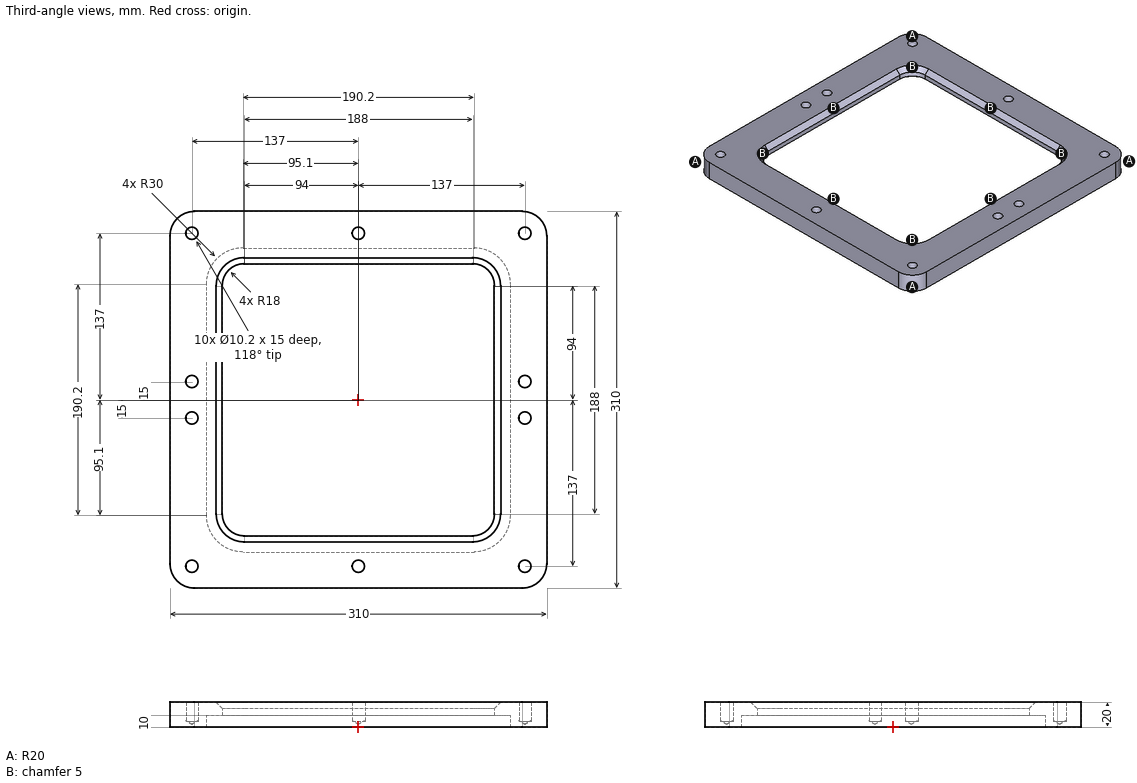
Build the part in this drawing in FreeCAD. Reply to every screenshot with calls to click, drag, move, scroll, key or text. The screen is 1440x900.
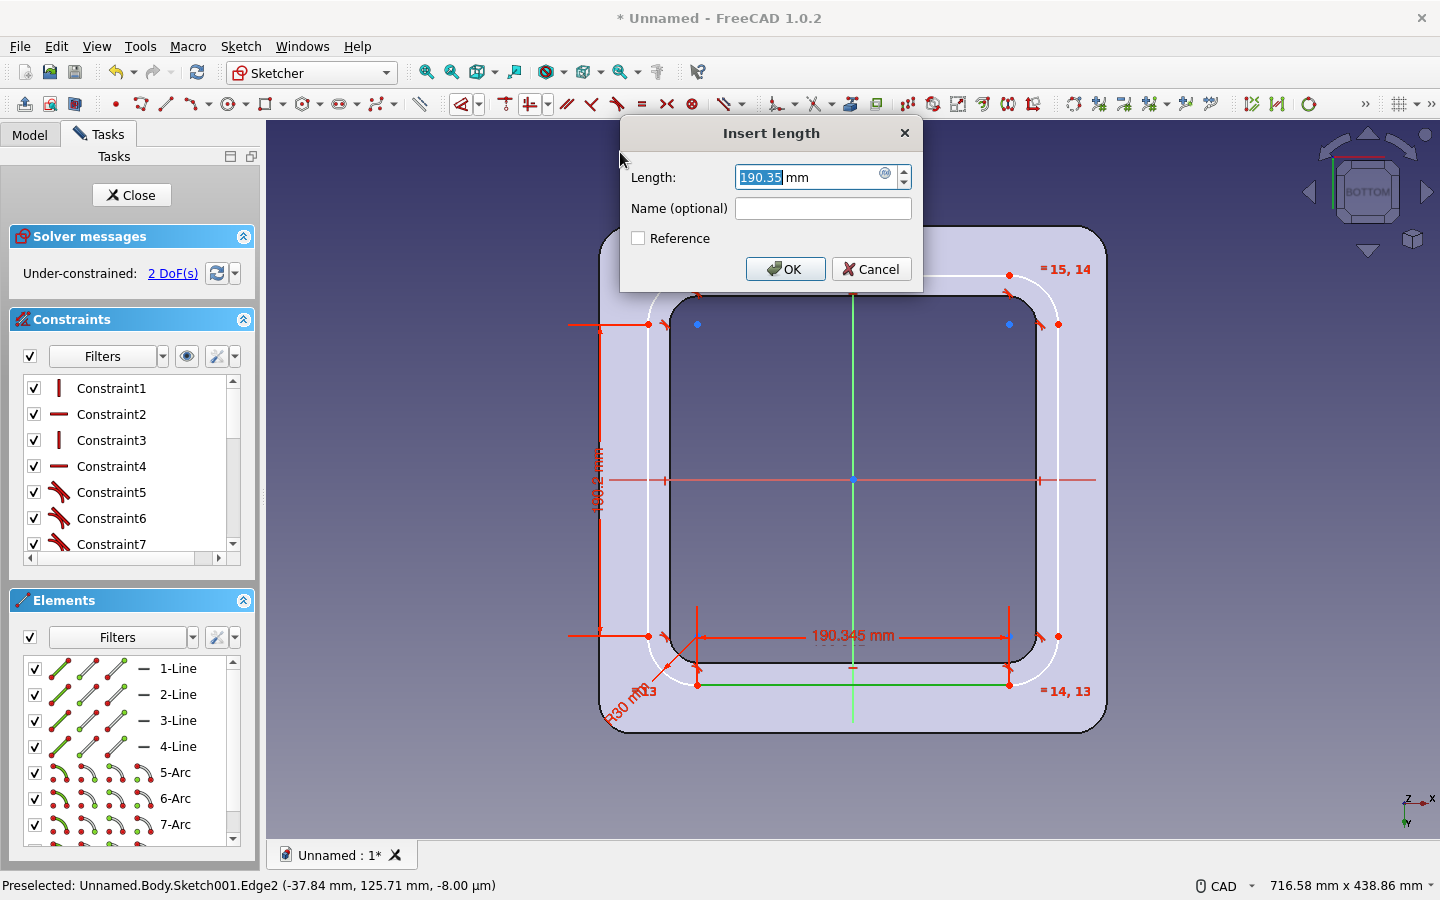
text(190.2)
key(Return)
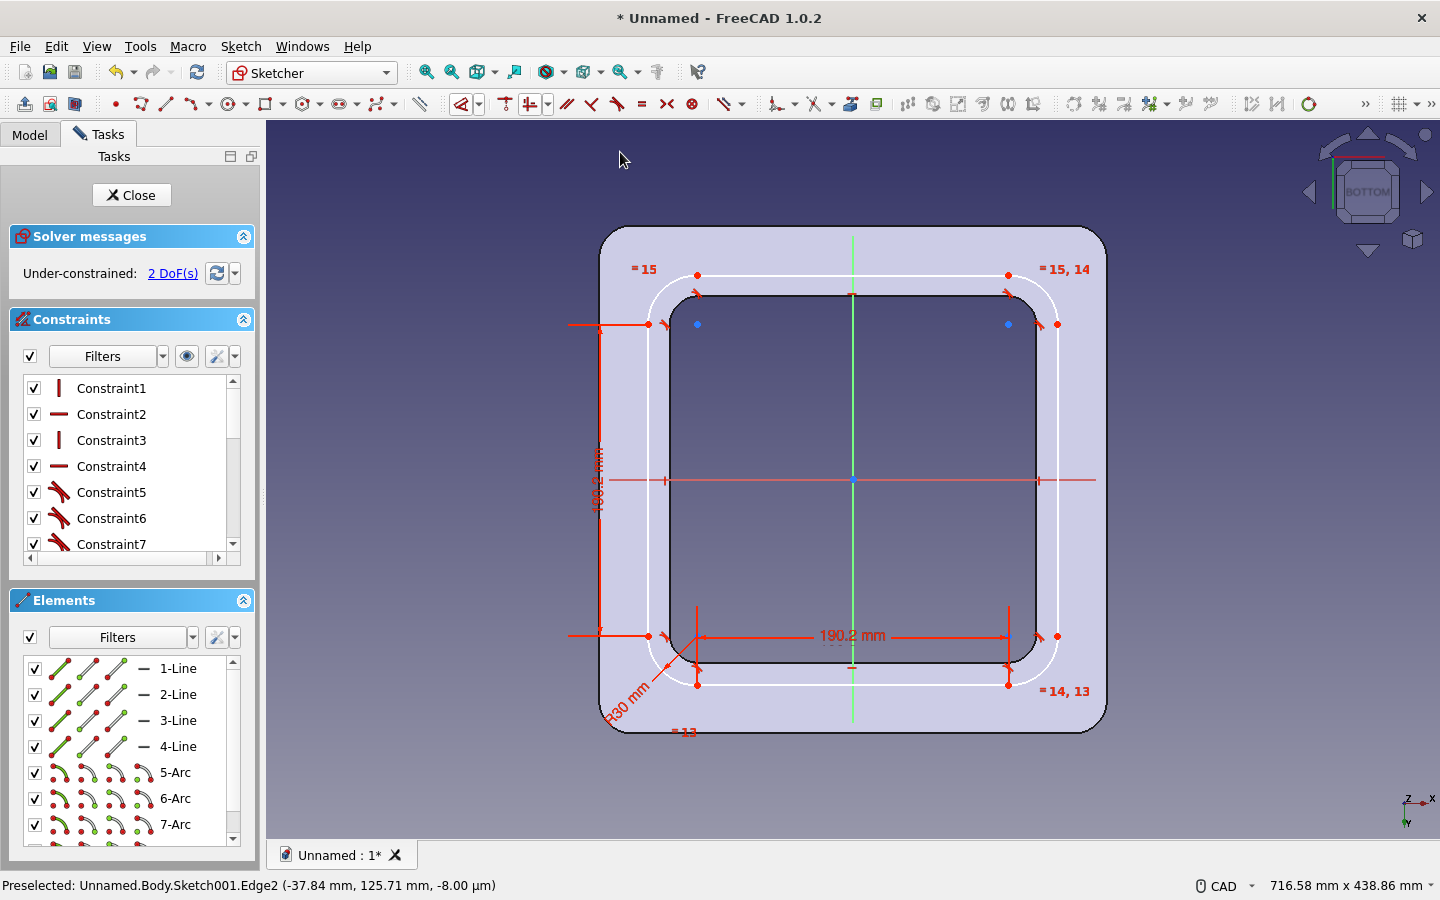
click(648, 325)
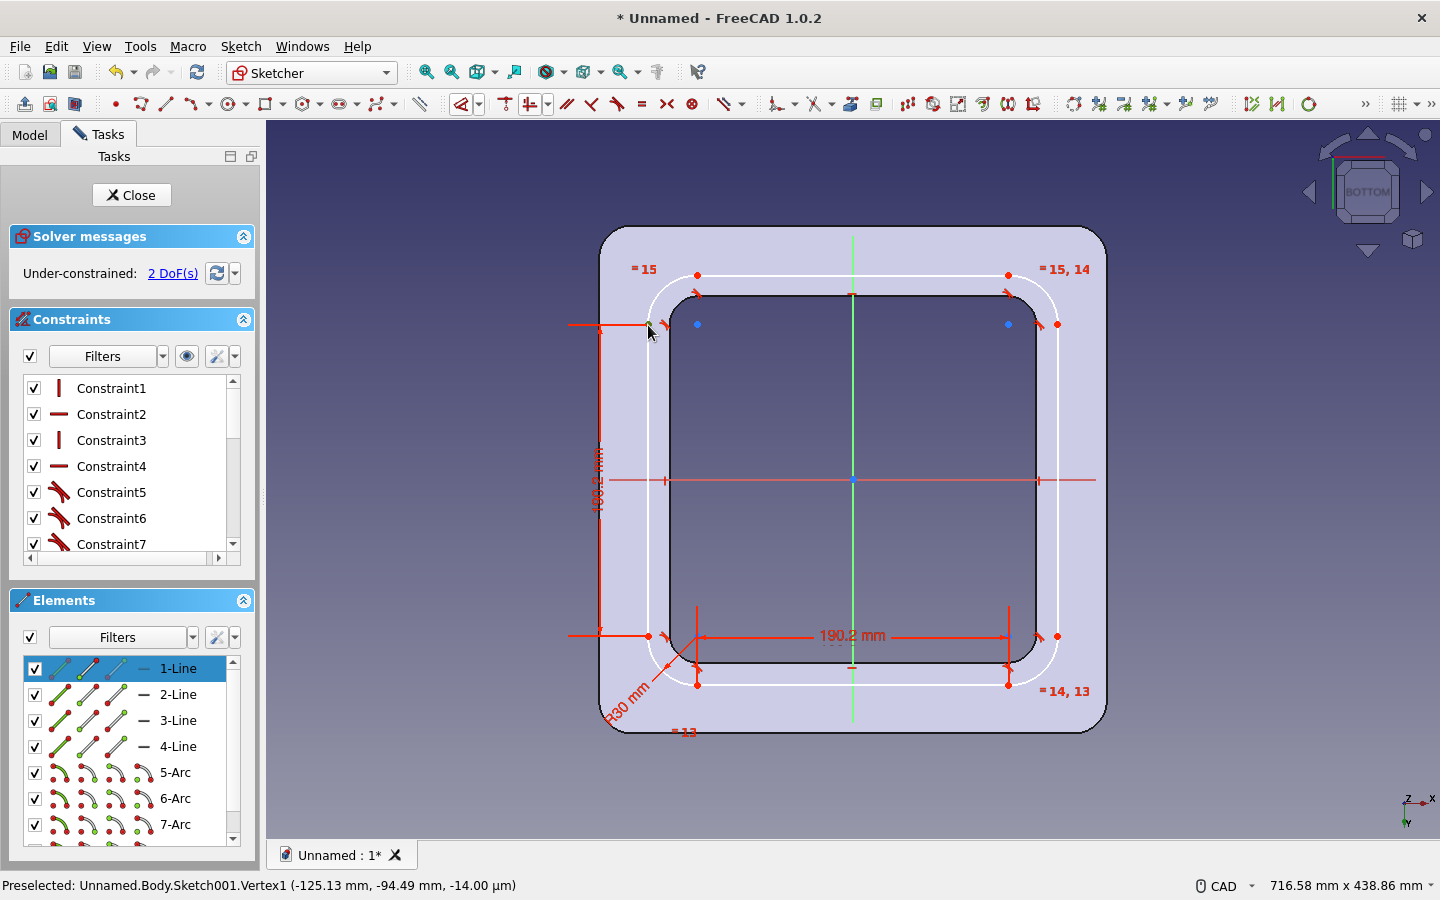
click(478, 104)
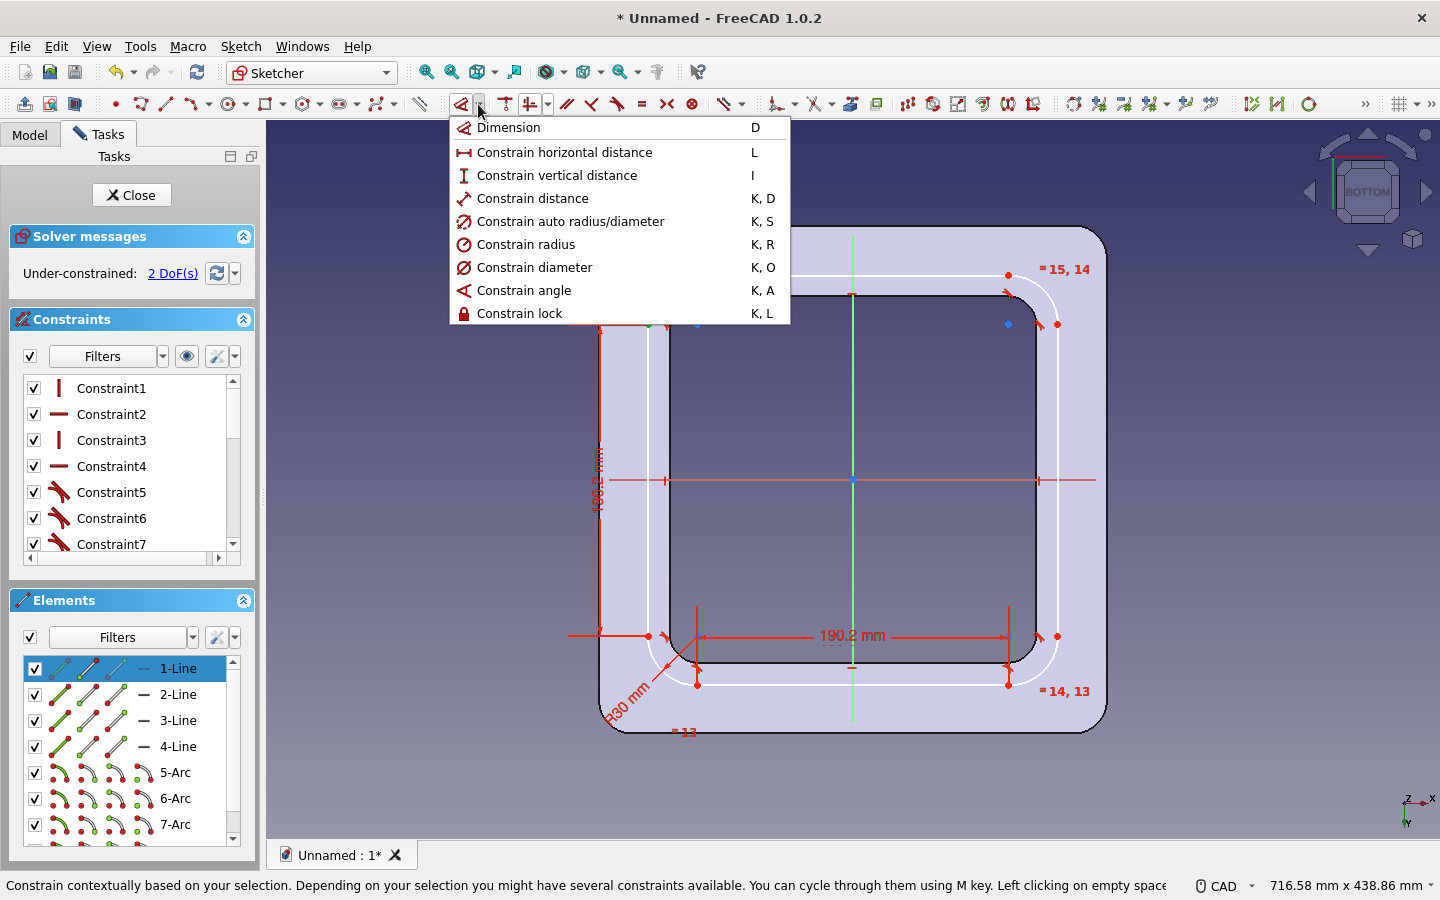
click(620, 176)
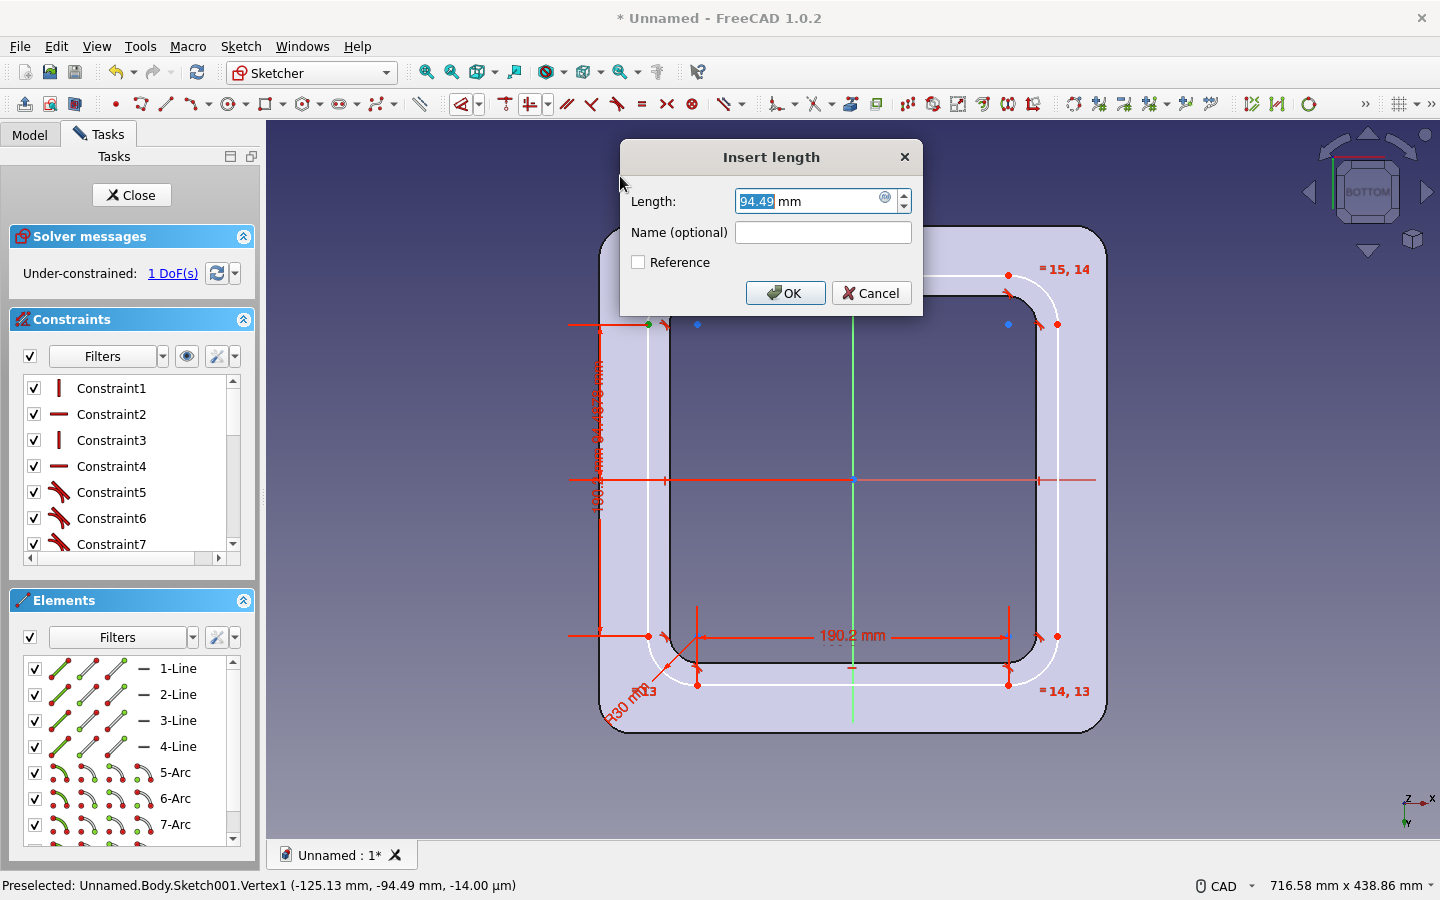
text(95.1)
key(Return)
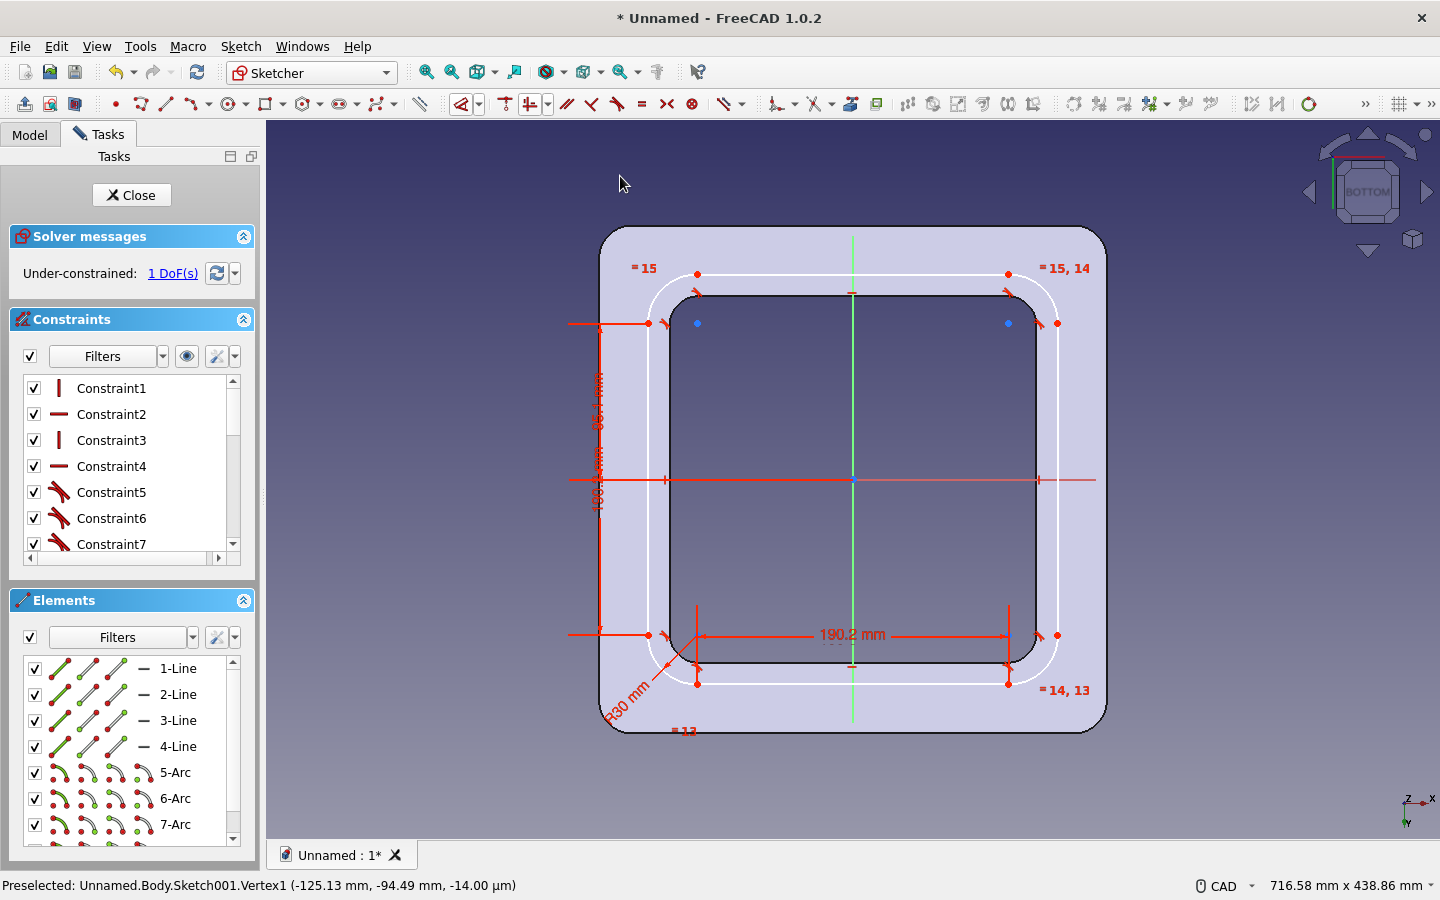
click(697, 684)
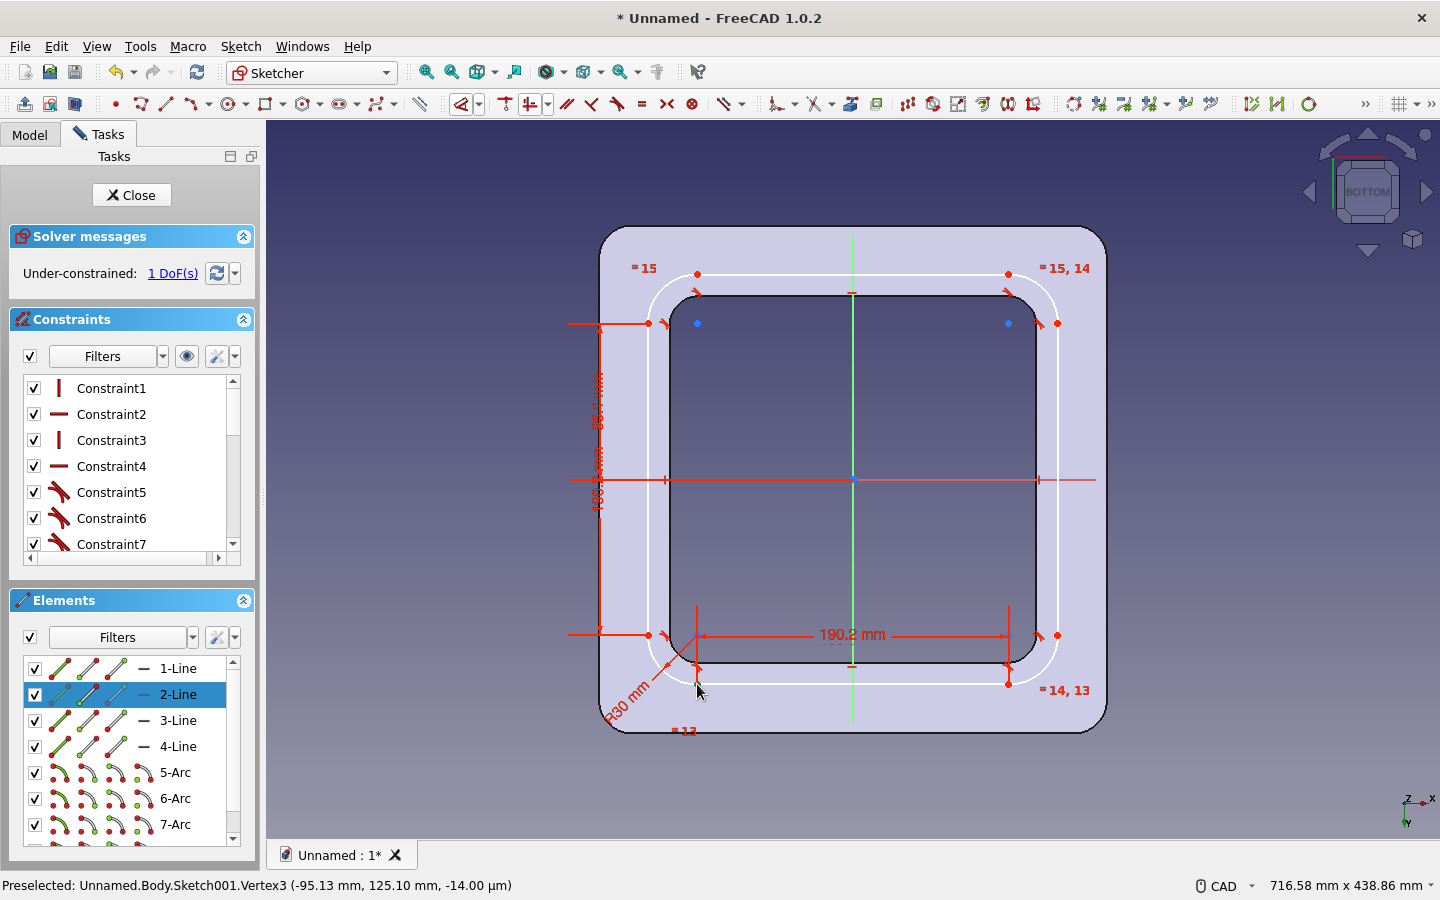
click(478, 104)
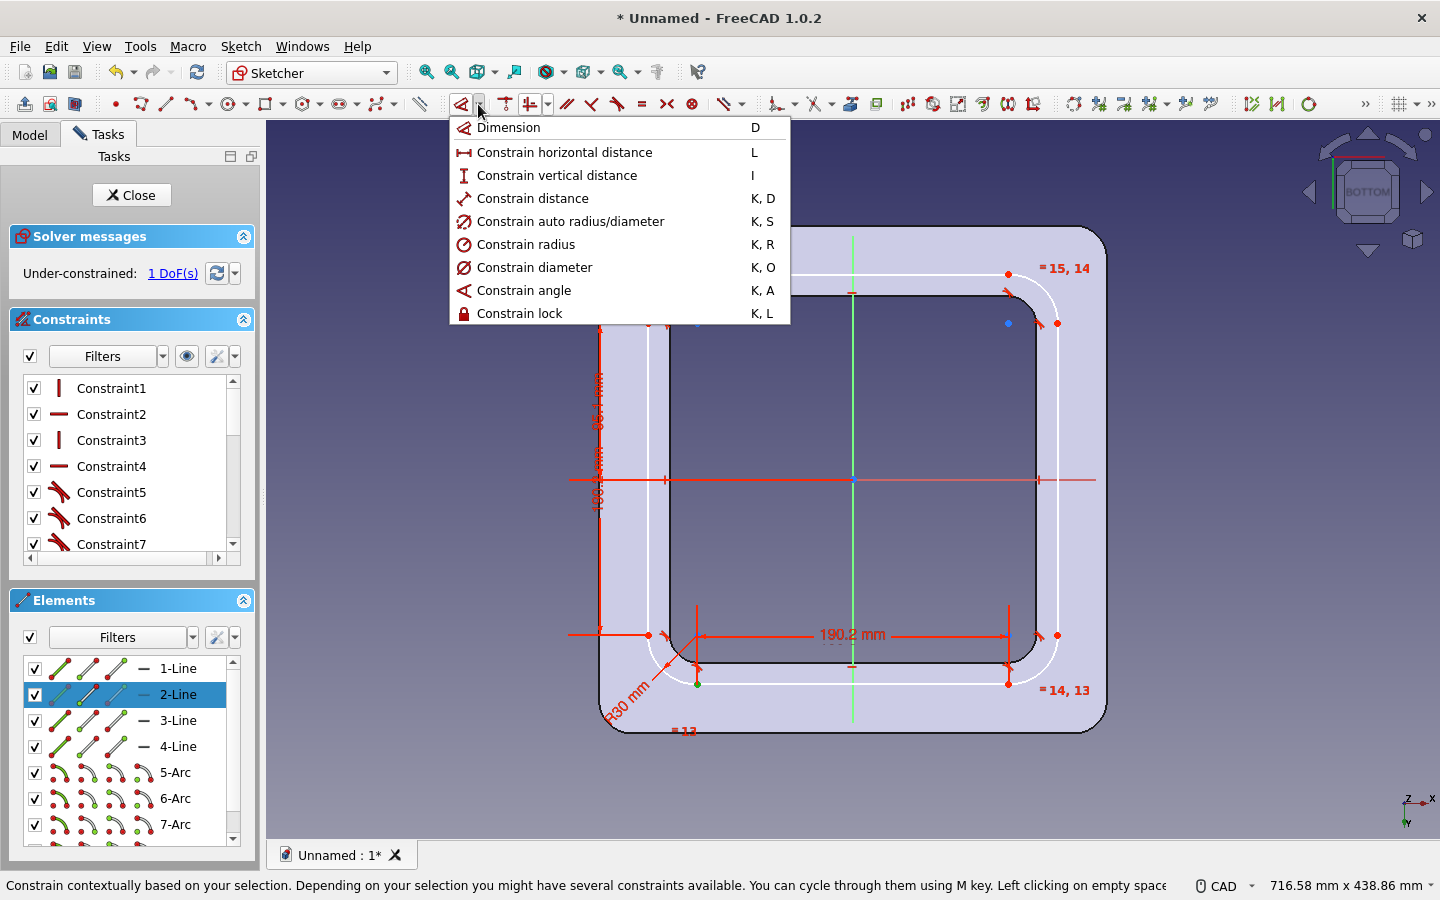
click(620, 152)